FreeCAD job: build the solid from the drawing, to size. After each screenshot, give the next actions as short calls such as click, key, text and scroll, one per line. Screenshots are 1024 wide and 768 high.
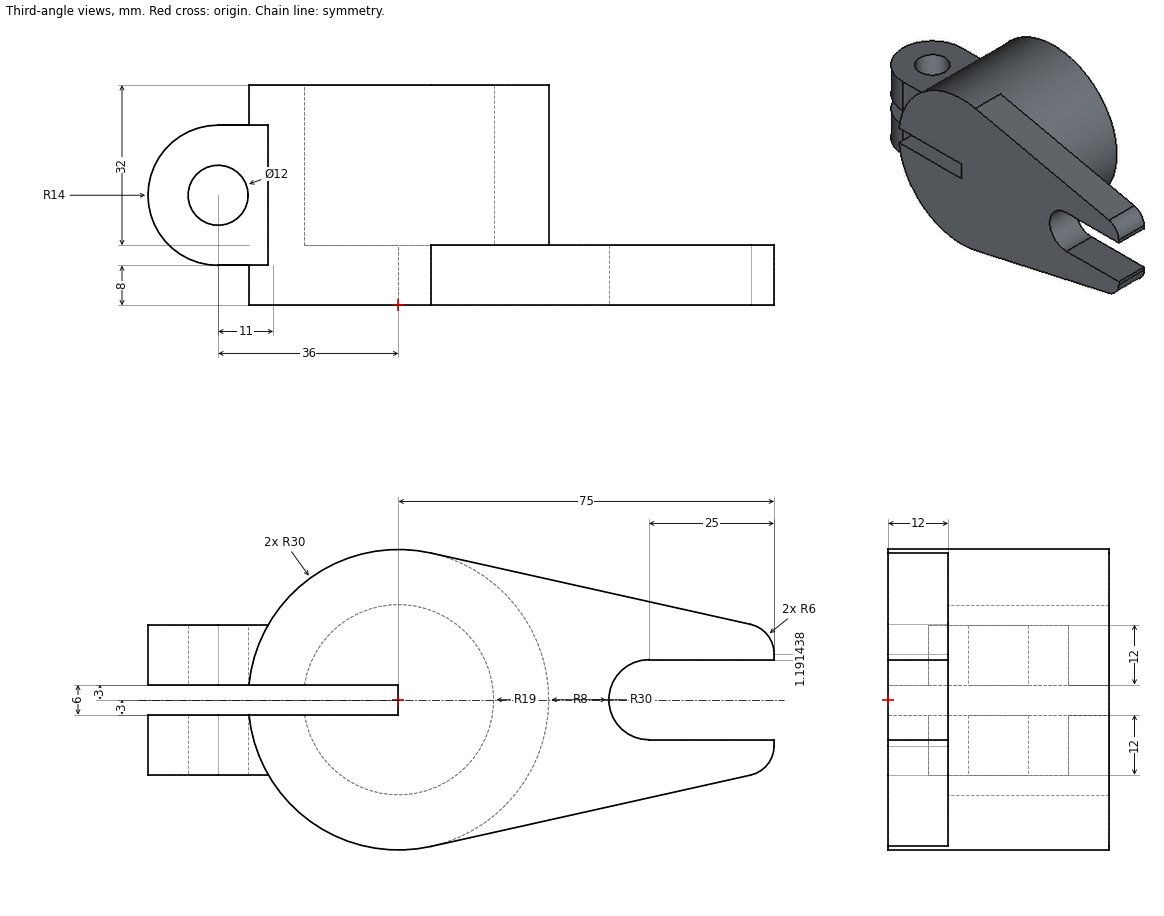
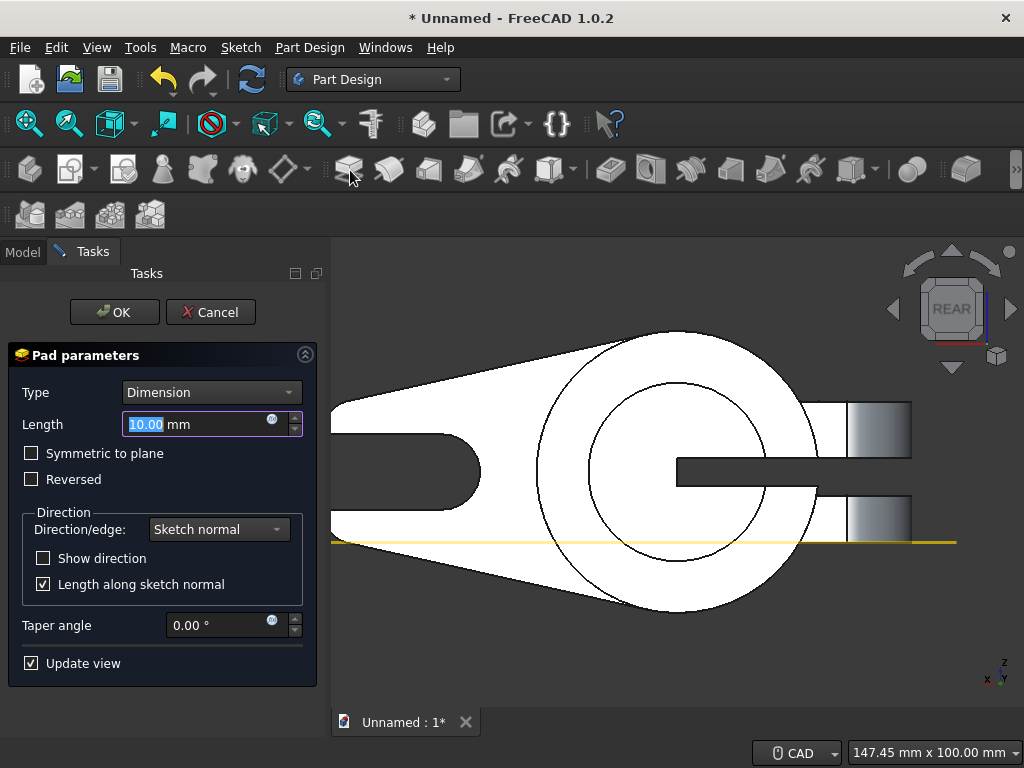
text(12)
key(Tab)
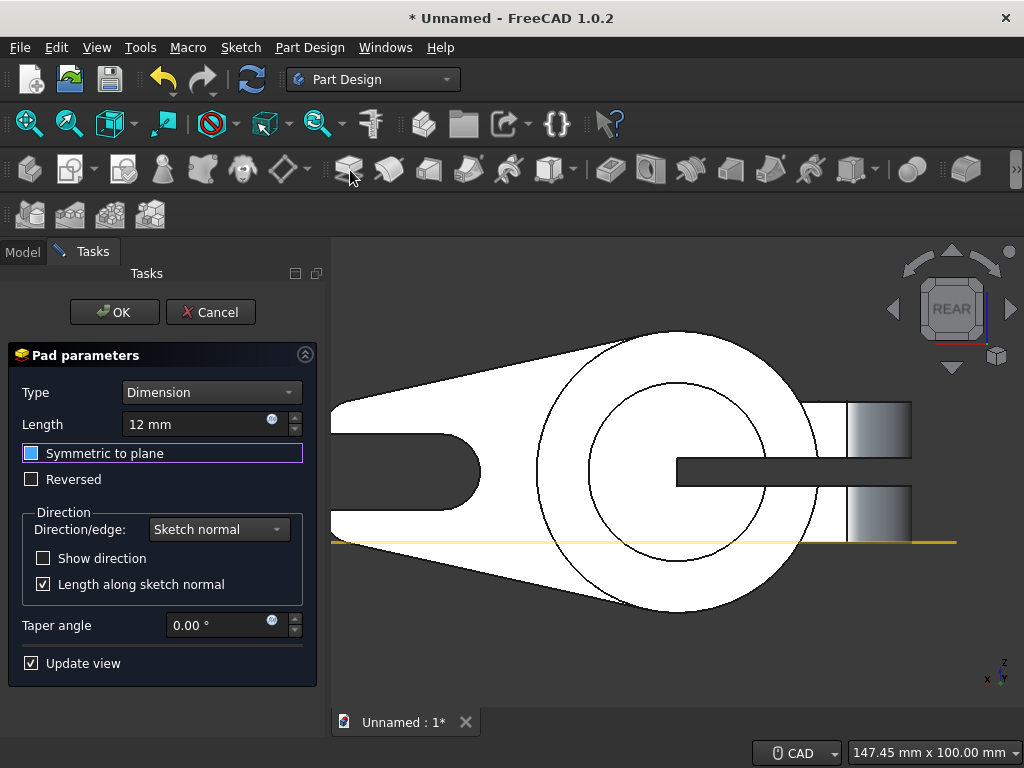
click(115, 312)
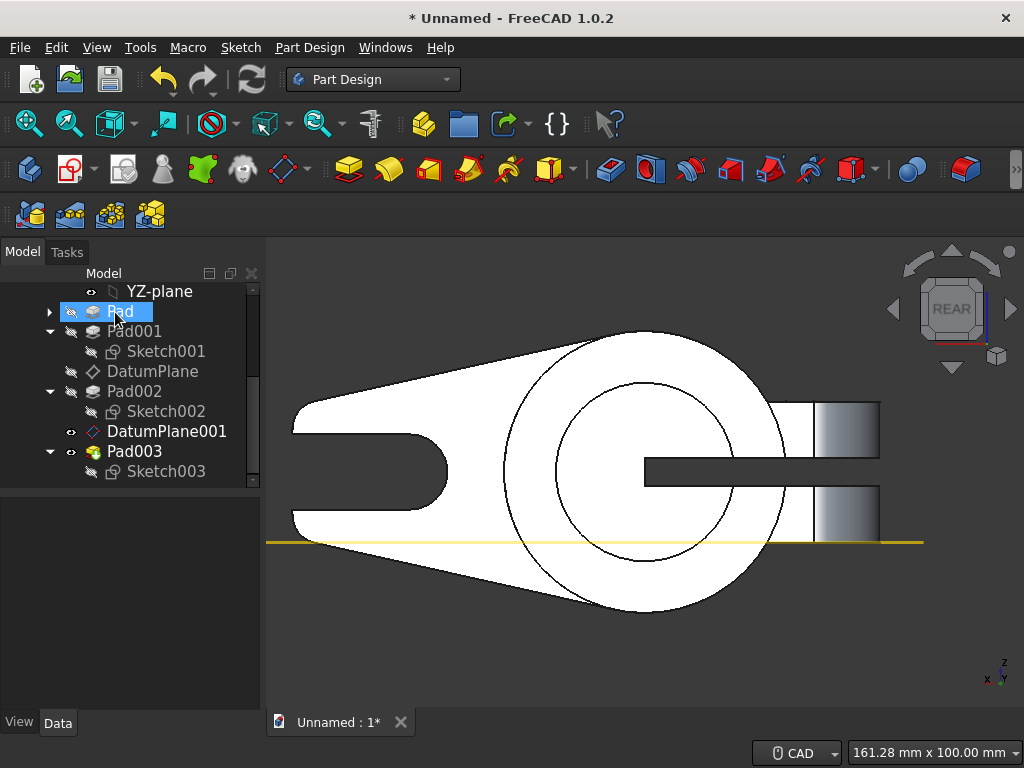
click(116, 432)
key(space)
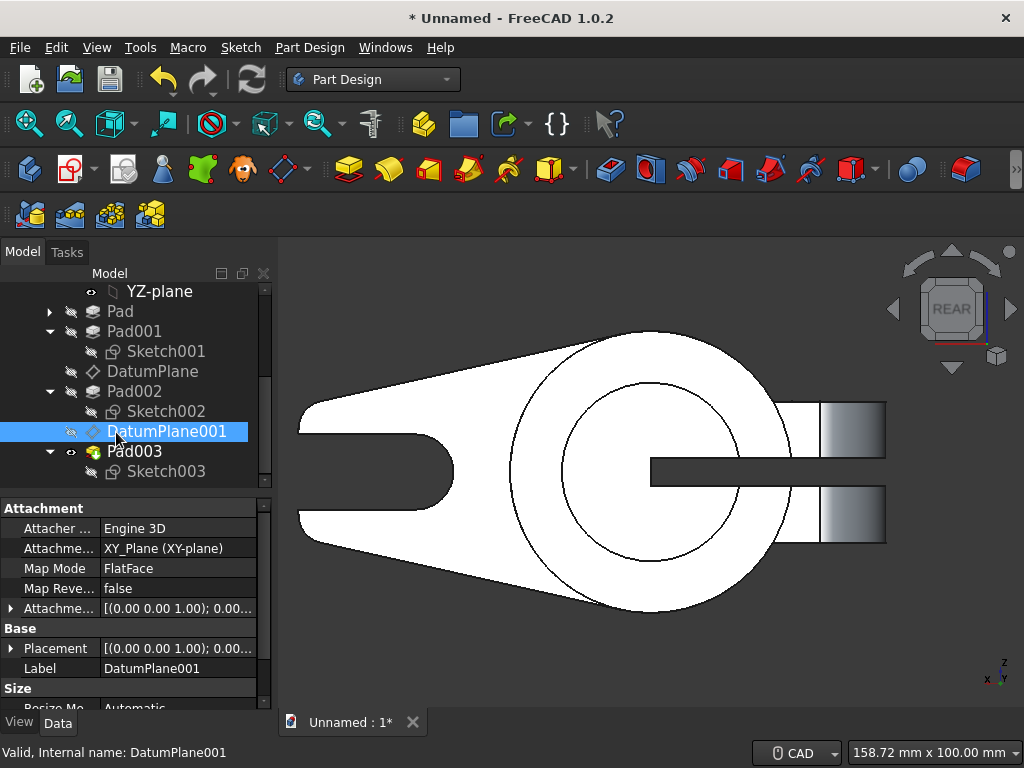
key(0)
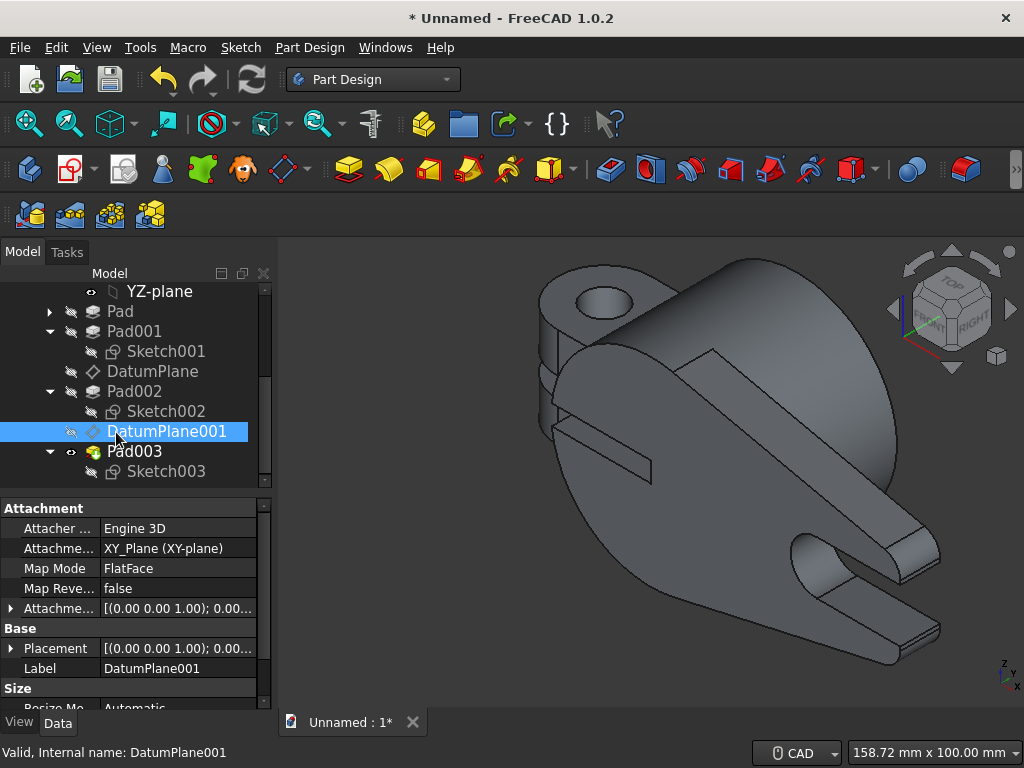
key(v)
key(f)